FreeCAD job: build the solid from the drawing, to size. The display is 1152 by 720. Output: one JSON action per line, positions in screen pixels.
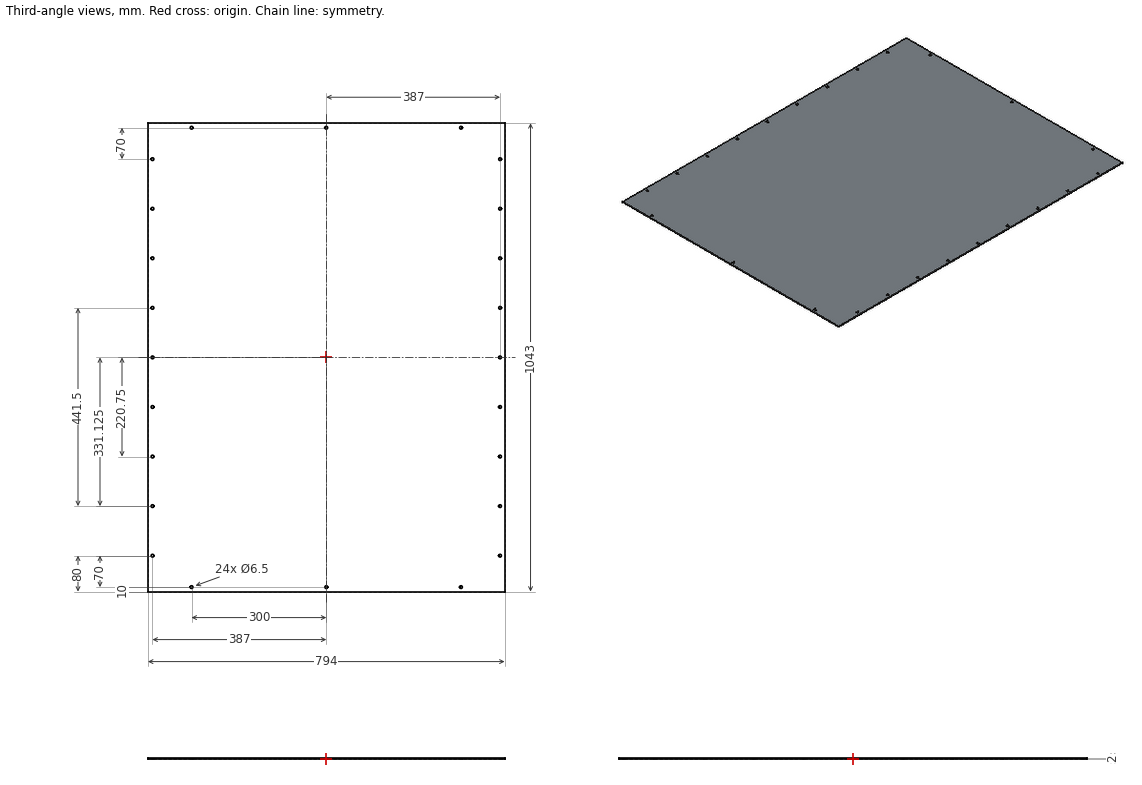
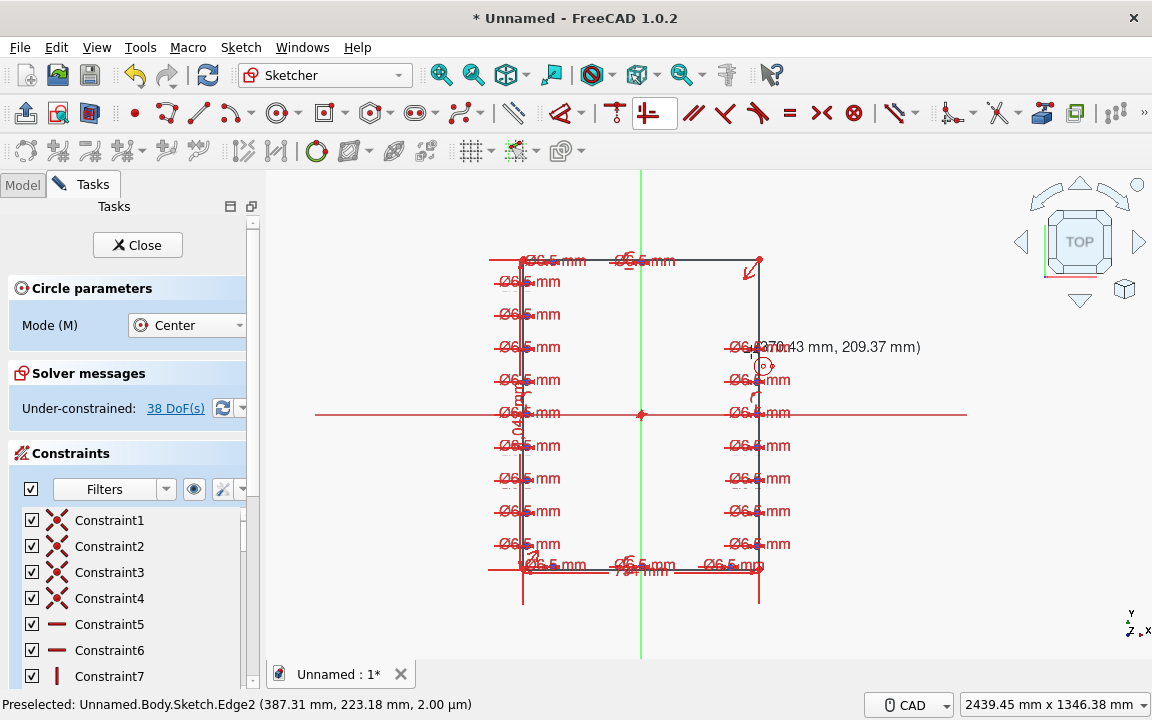
{"action": "scroll", "coordinate": [756, 316], "scroll_direction": "up", "scroll_amount": 16}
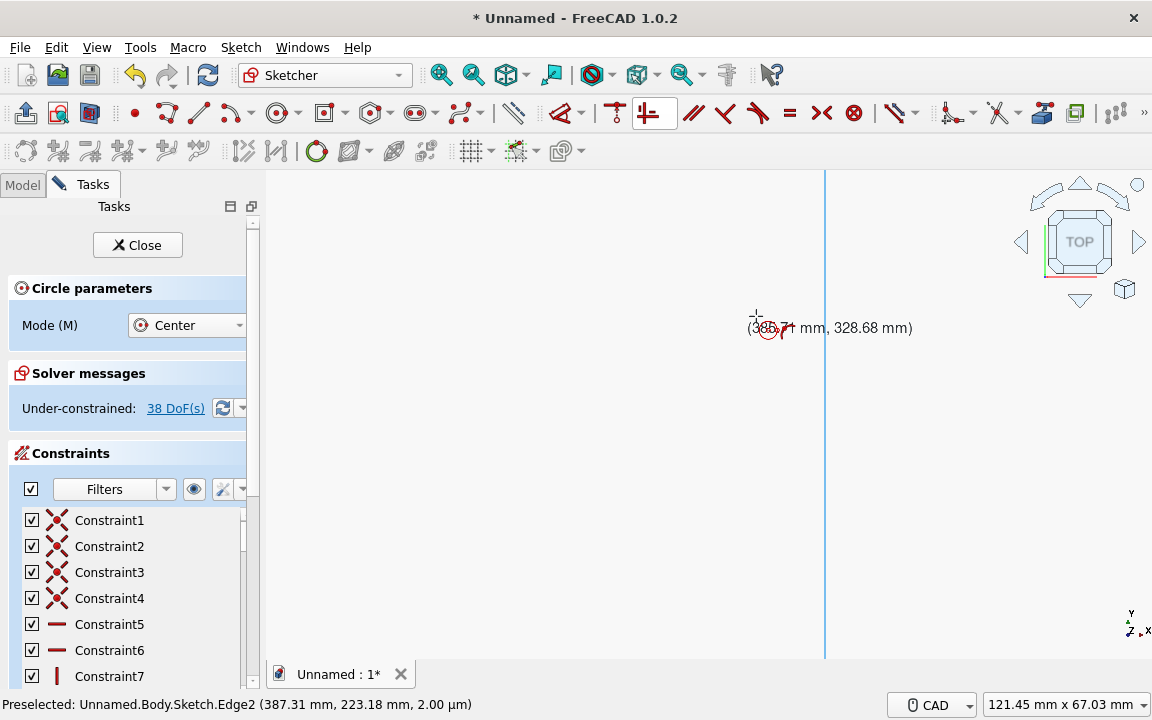
{"action": "scroll", "coordinate": [783, 293], "scroll_direction": "down", "scroll_amount": 15}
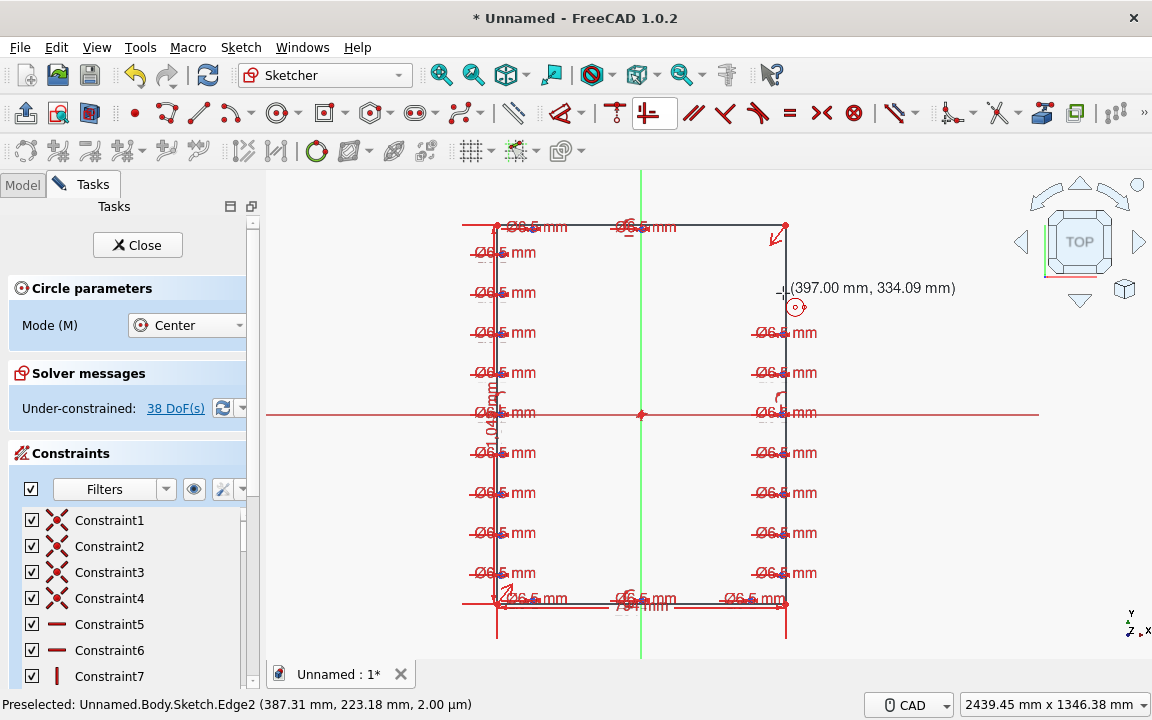
{"action": "scroll", "coordinate": [782, 294], "scroll_direction": "up", "scroll_amount": 8}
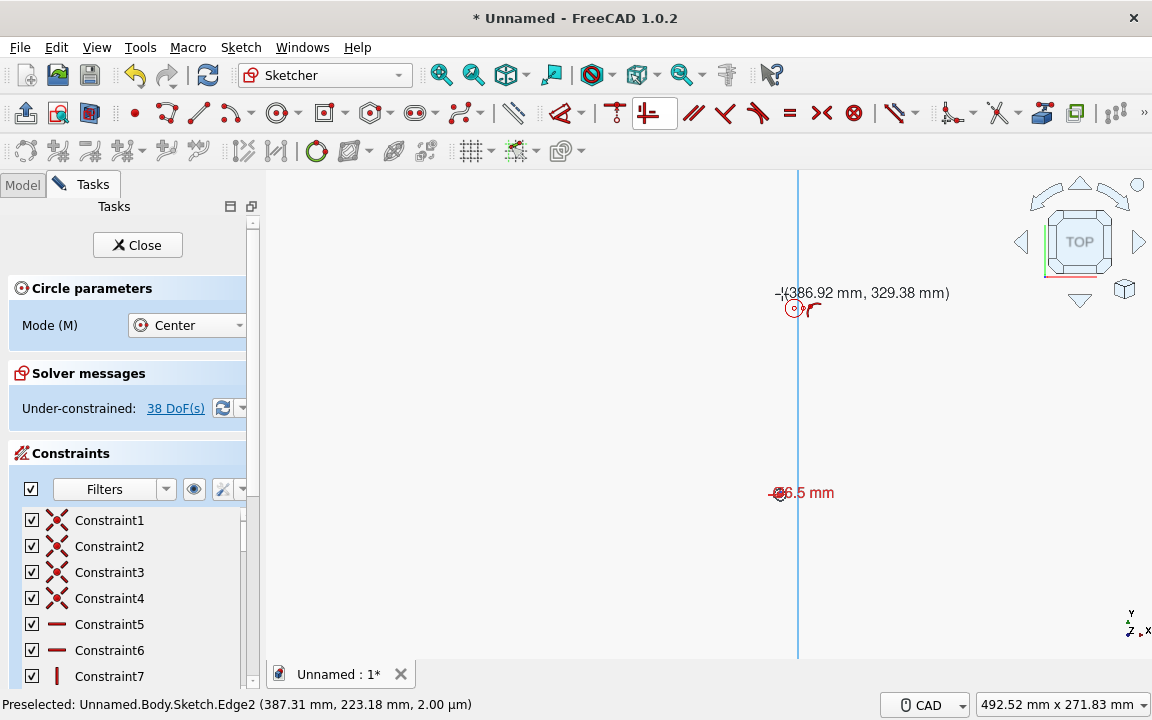
{"action": "left_click", "coordinate": [780, 295]}
{"action": "mouse_move", "coordinate": [776, 291]}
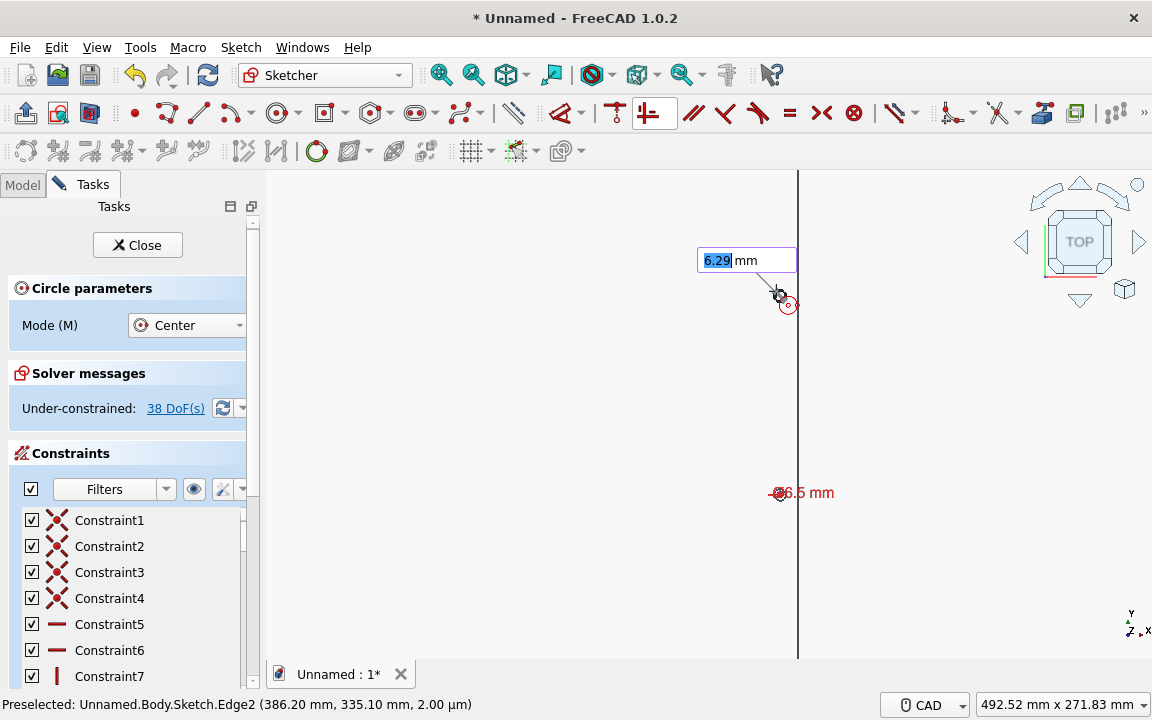
{"action": "type", "text": "6.5"}
{"action": "key", "text": "Return"}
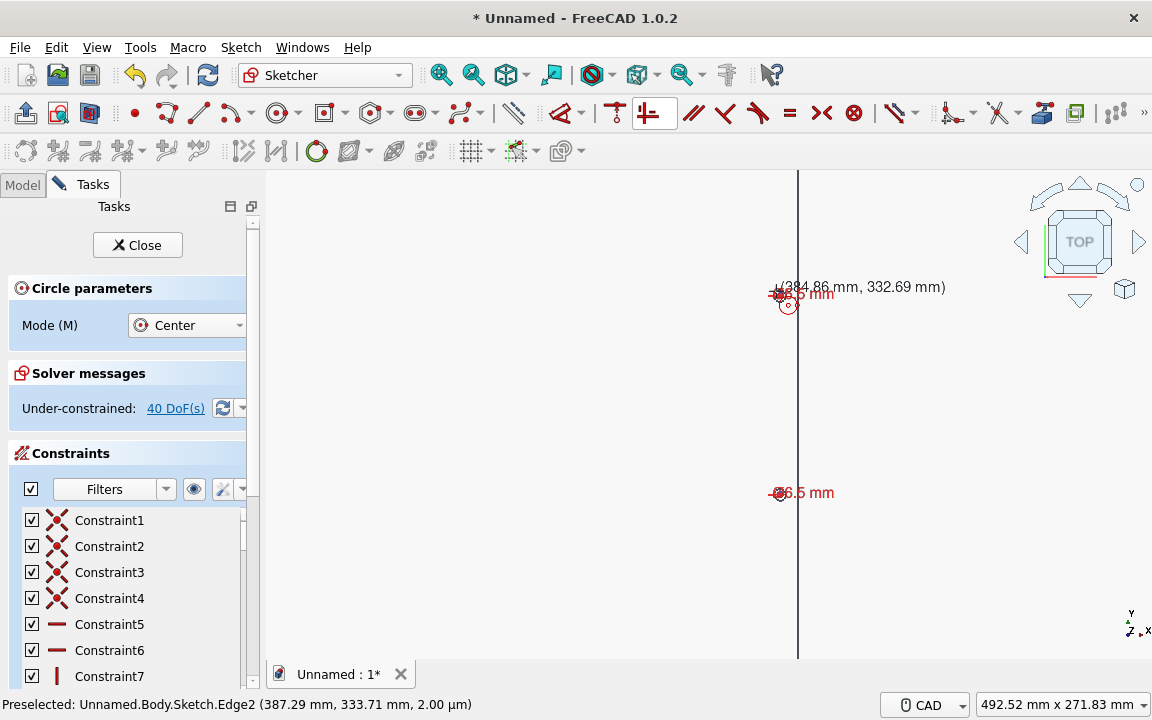
{"action": "scroll", "coordinate": [751, 320], "scroll_direction": "down", "scroll_amount": 9}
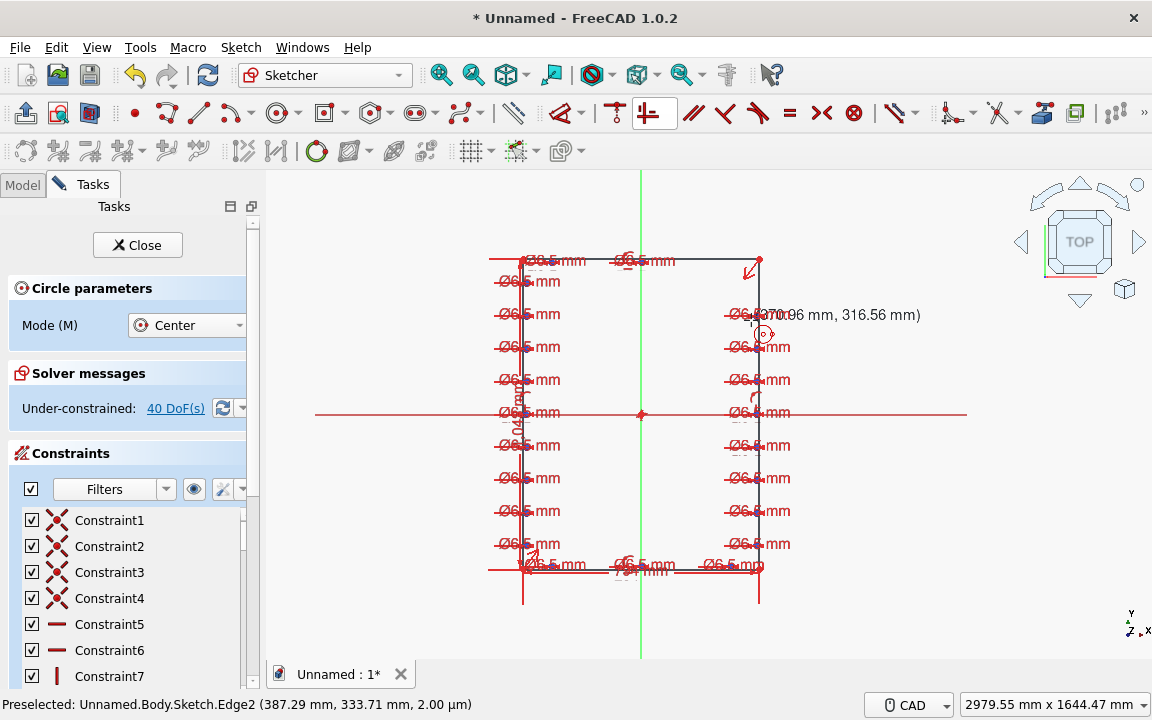
{"action": "scroll", "coordinate": [756, 283], "scroll_direction": "up", "scroll_amount": 16}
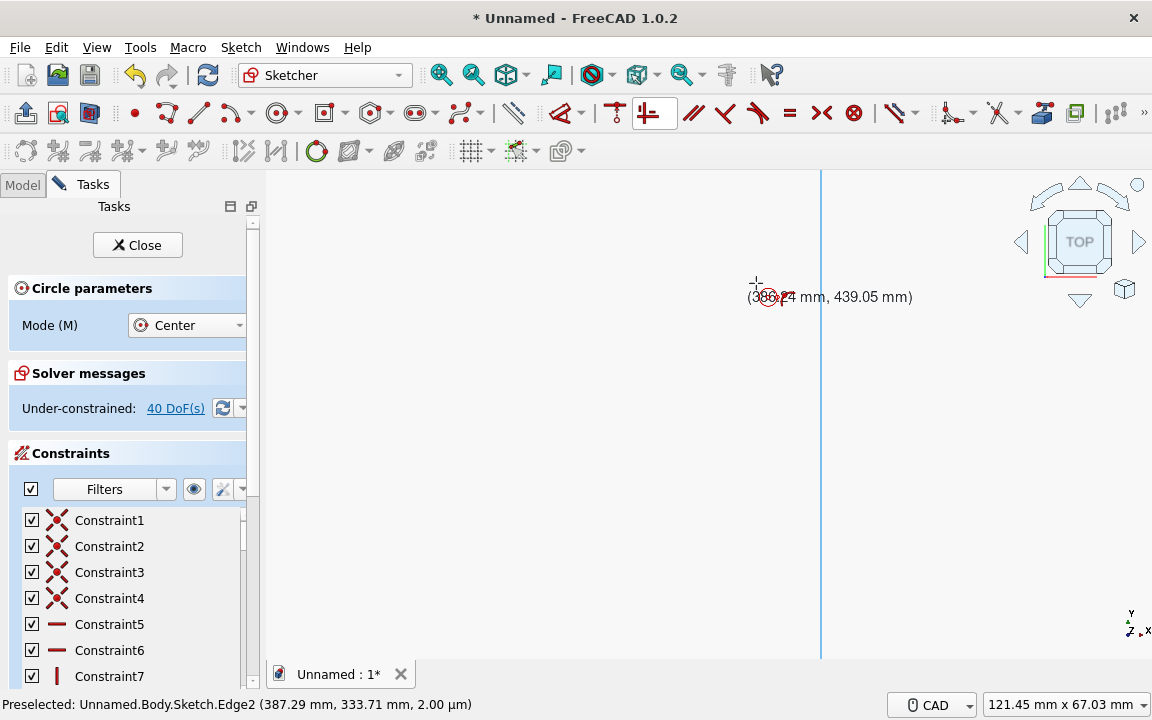
{"action": "scroll", "coordinate": [783, 253], "scroll_direction": "down", "scroll_amount": 15}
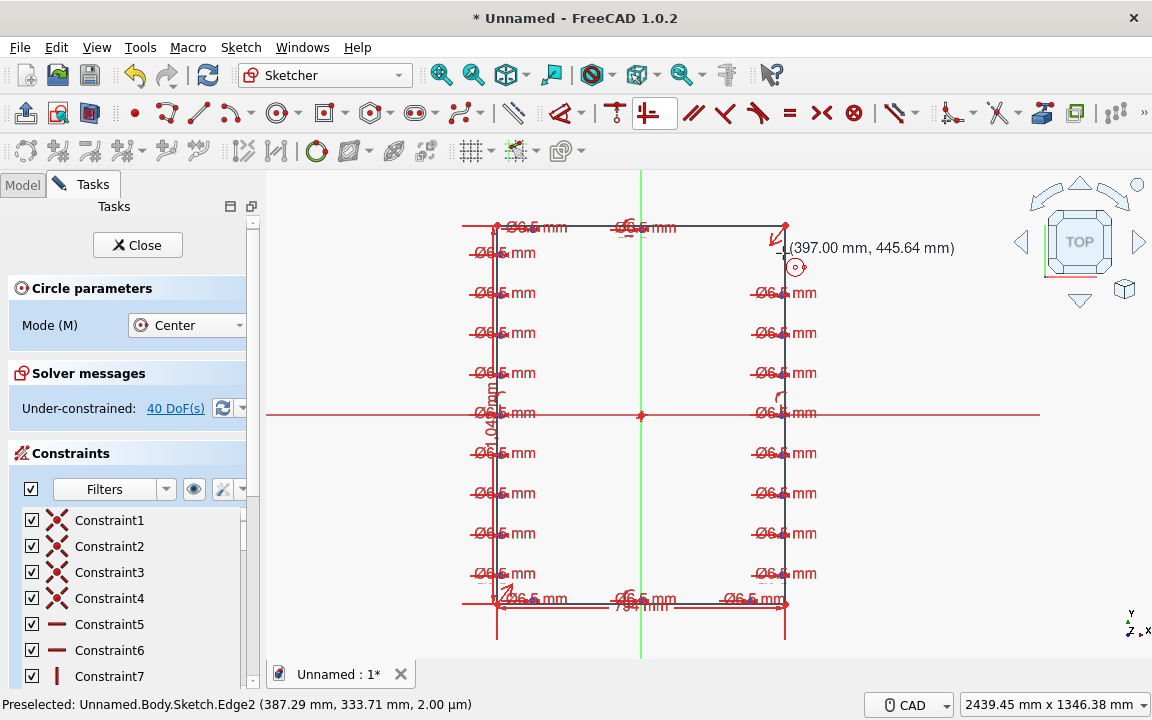
{"action": "scroll", "coordinate": [782, 255], "scroll_direction": "up", "scroll_amount": 8}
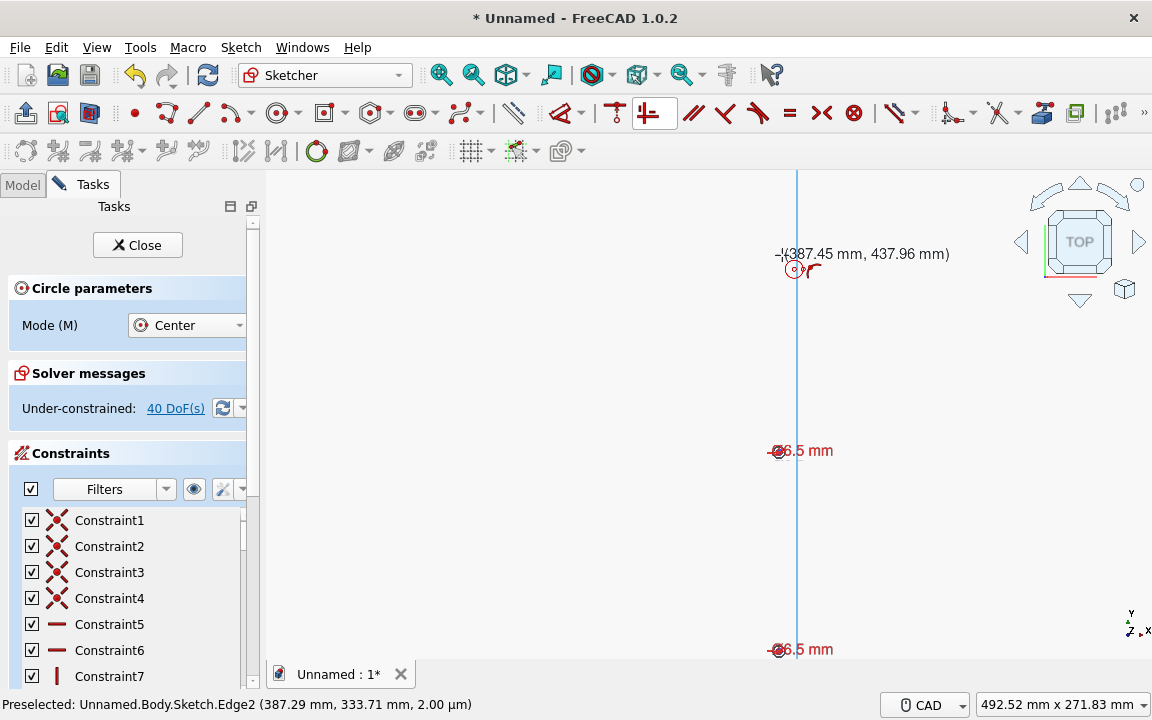
{"action": "left_click", "coordinate": [779, 253]}
{"action": "mouse_move", "coordinate": [775, 249]}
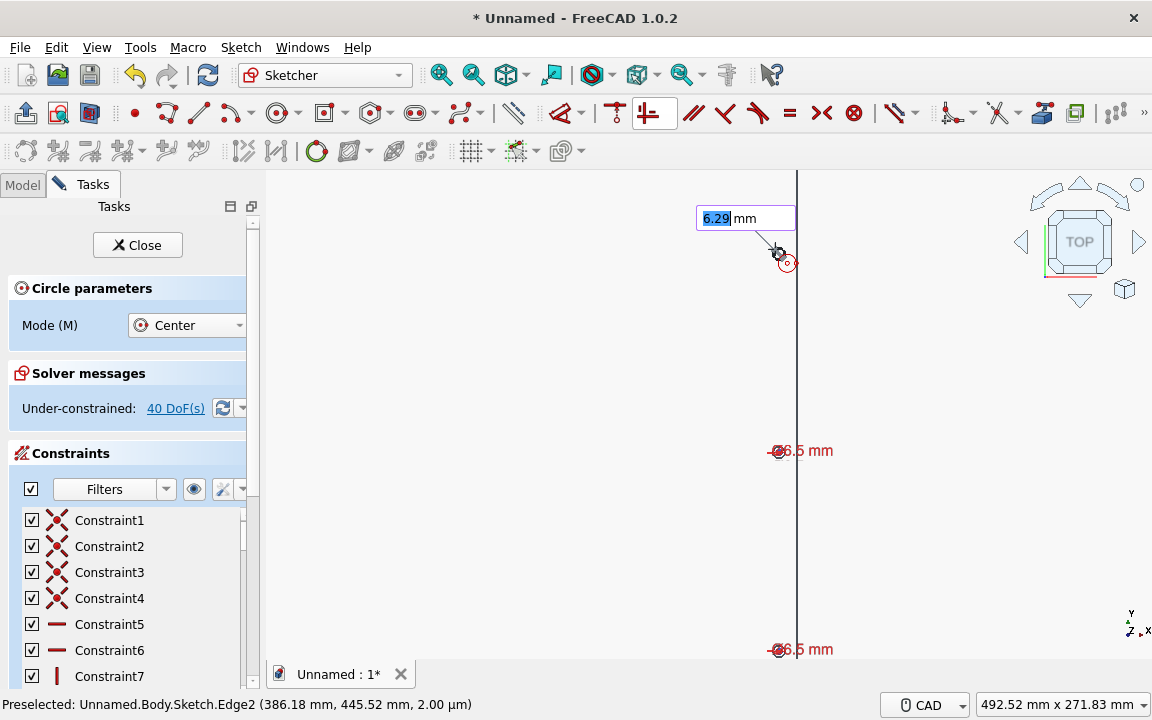
{"action": "type", "text": "6.5"}
{"action": "key", "text": "Return"}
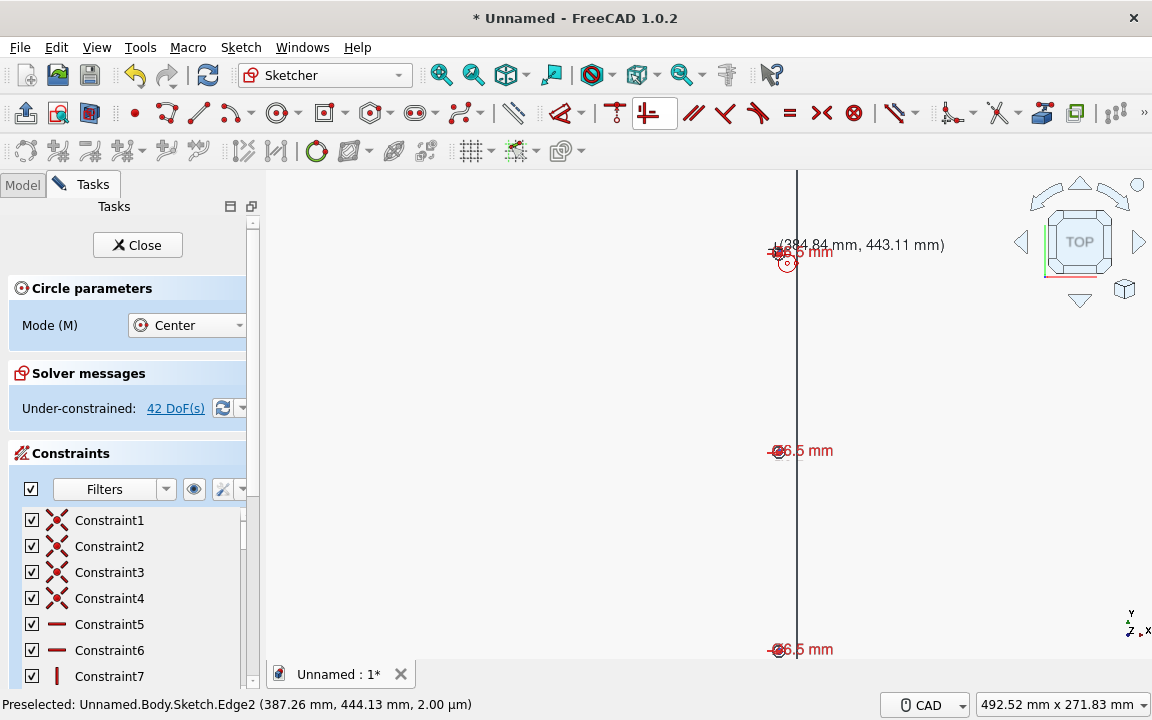
{"action": "scroll", "coordinate": [751, 289], "scroll_direction": "down", "scroll_amount": 9}